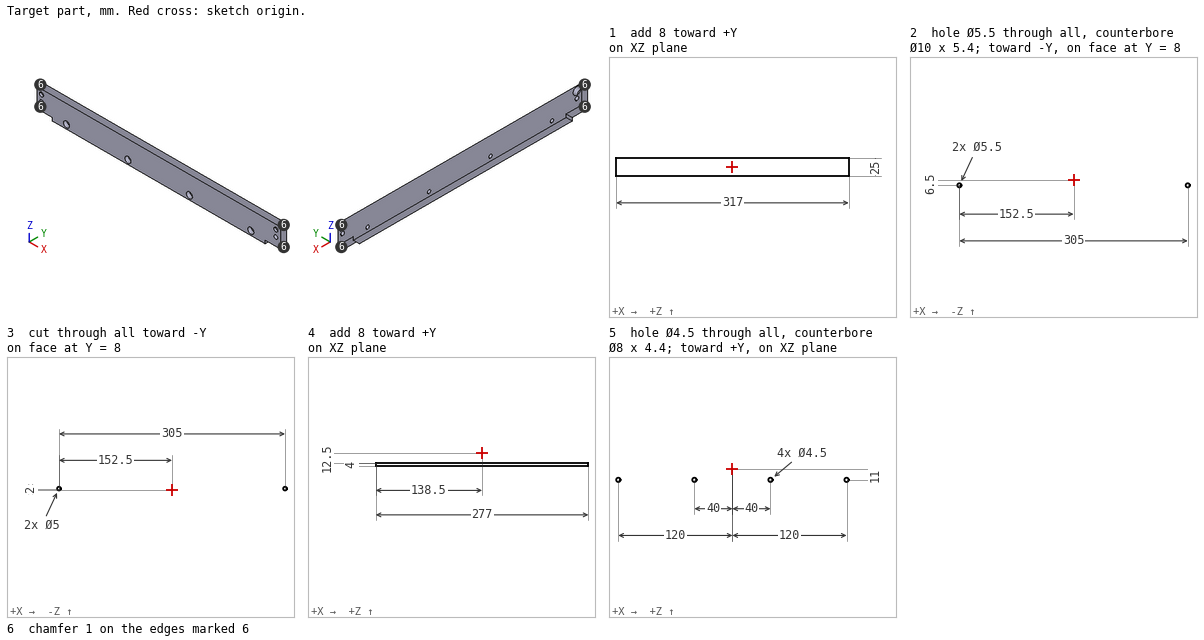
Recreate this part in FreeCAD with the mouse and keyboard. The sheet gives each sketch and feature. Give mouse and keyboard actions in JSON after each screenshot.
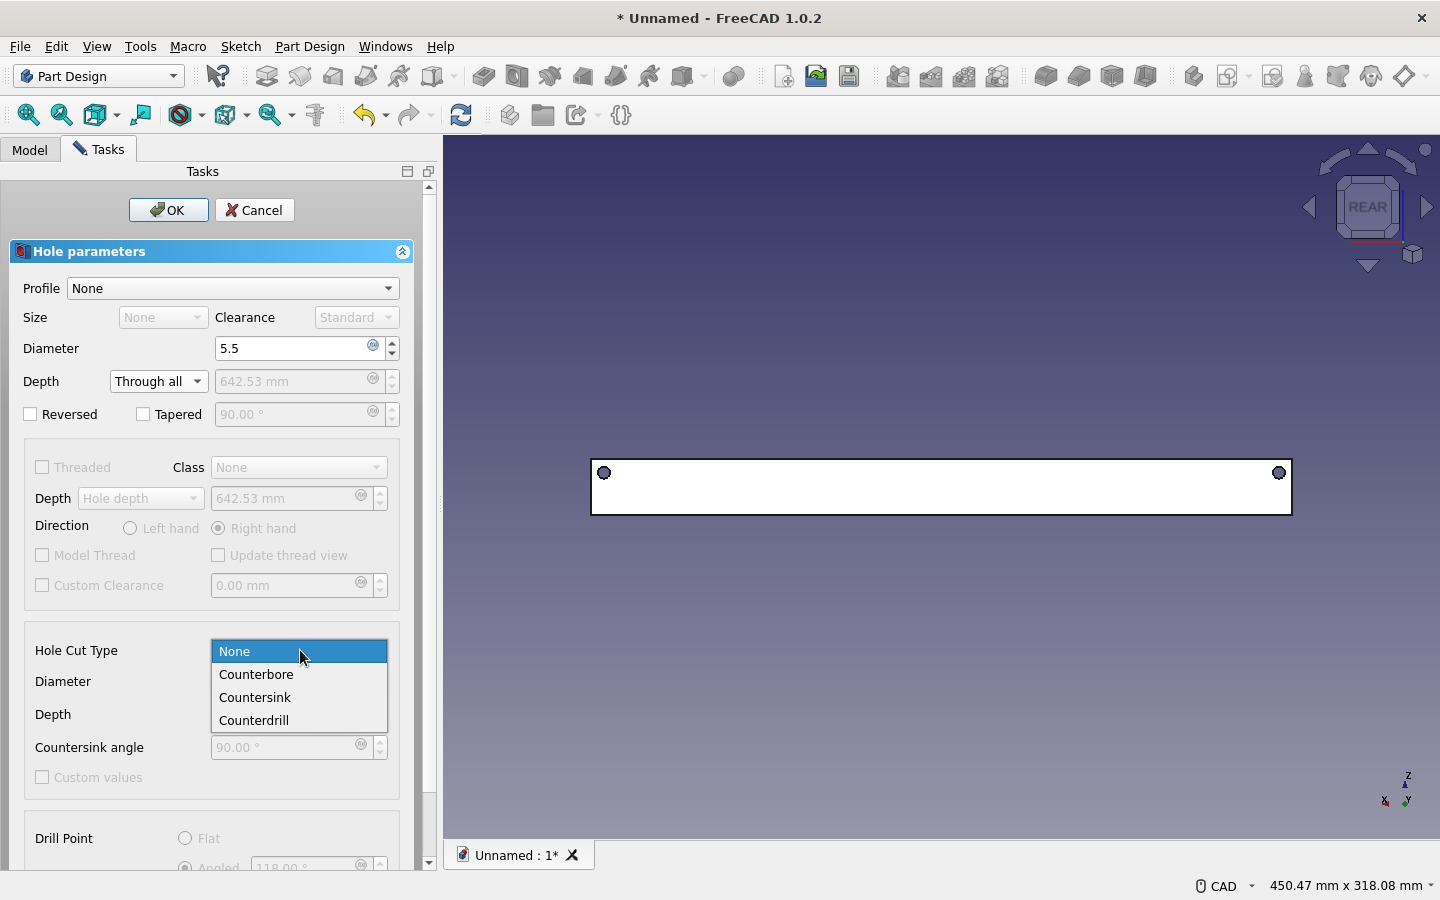
{"action": "left_click", "coordinate": [298, 674]}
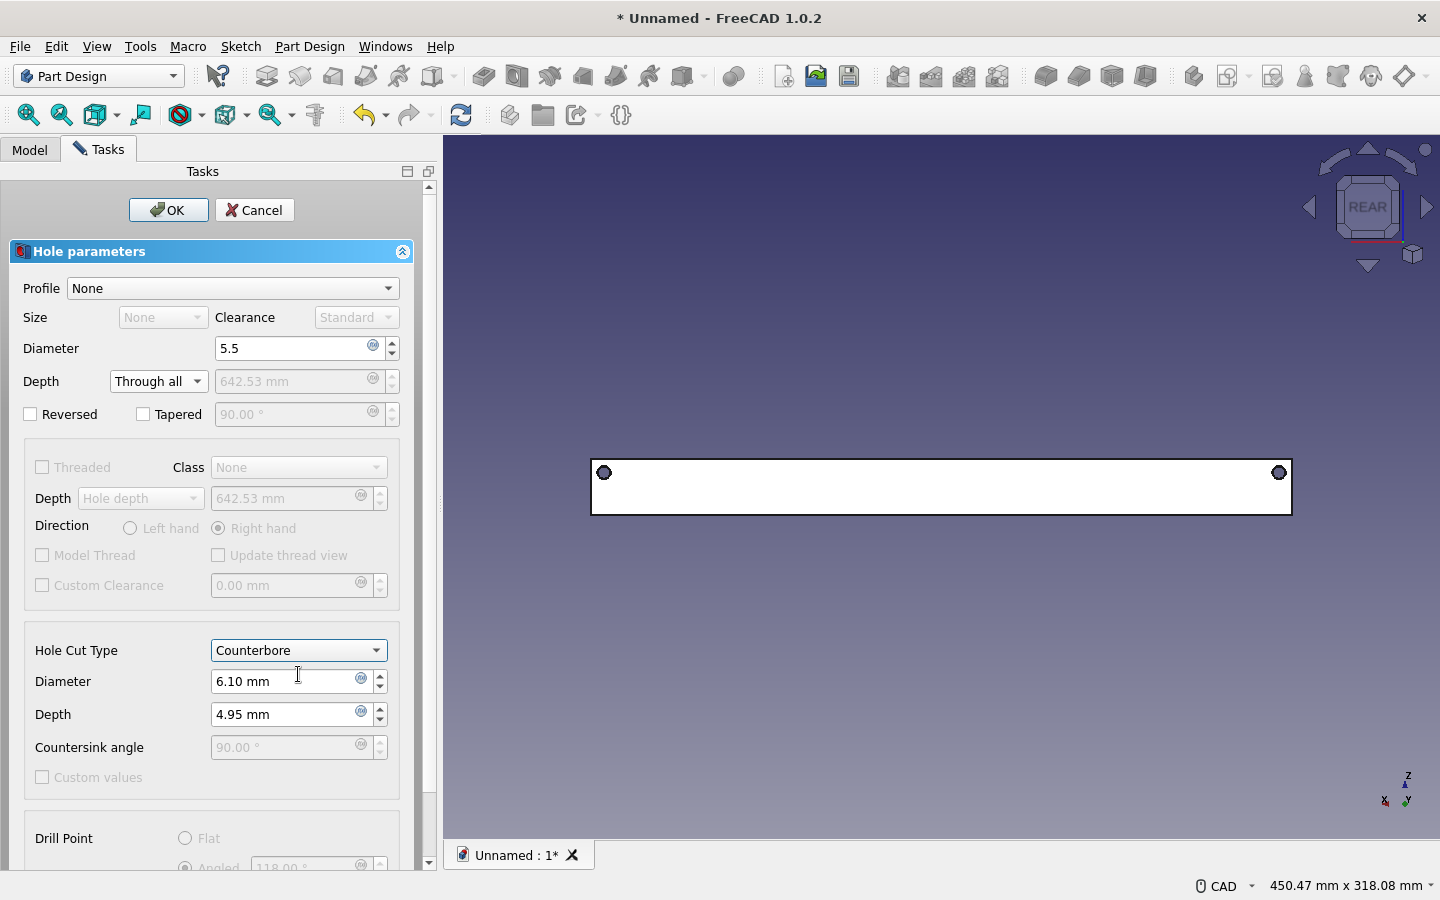
{"action": "triple_click", "coordinate": [292, 682]}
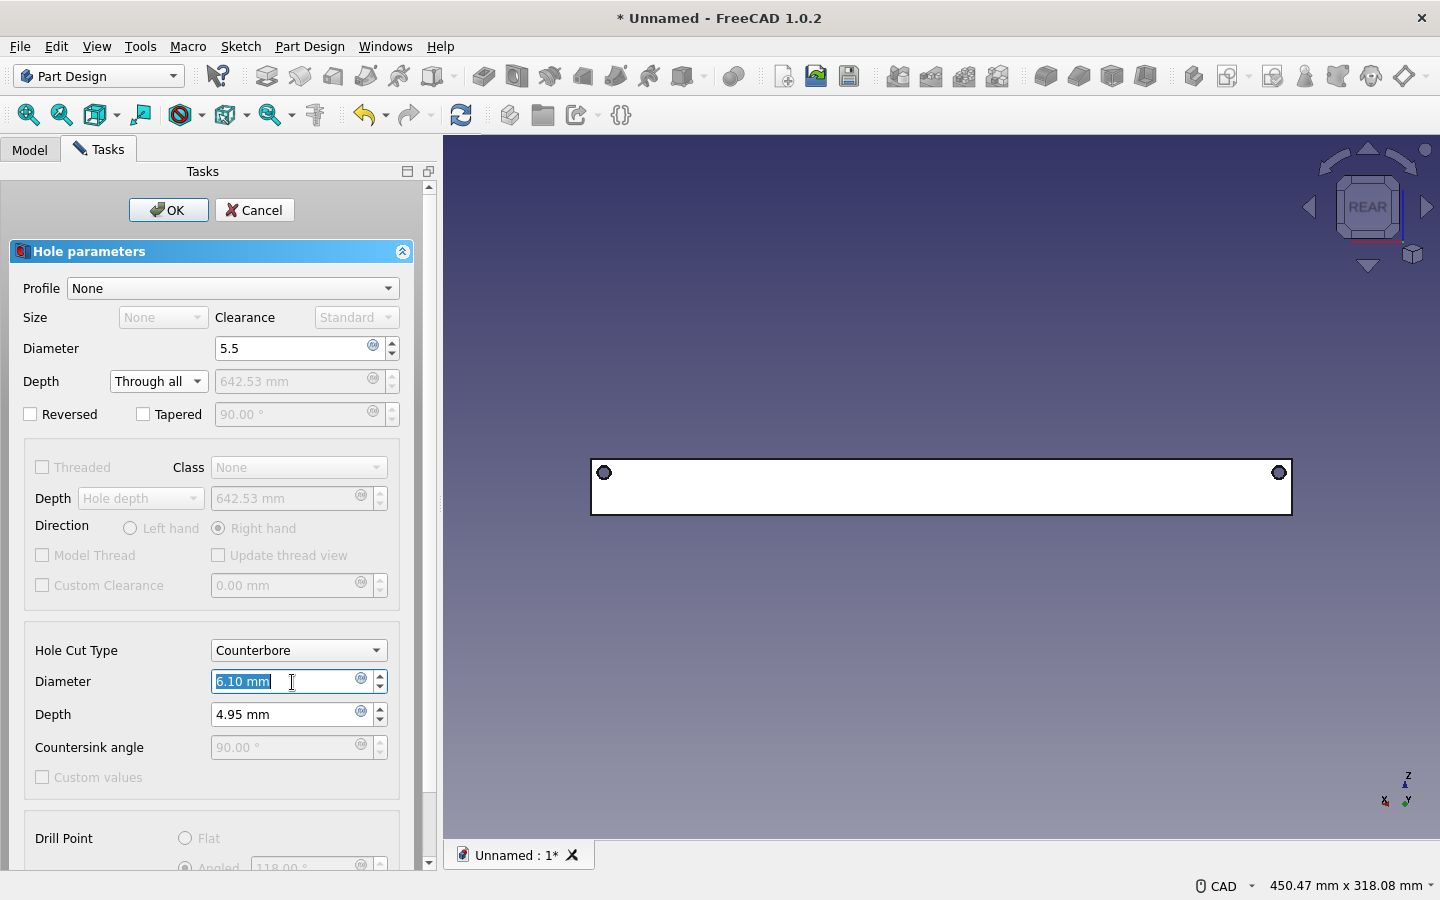
{"action": "type", "text": "10"}
{"action": "key", "text": "Tab"}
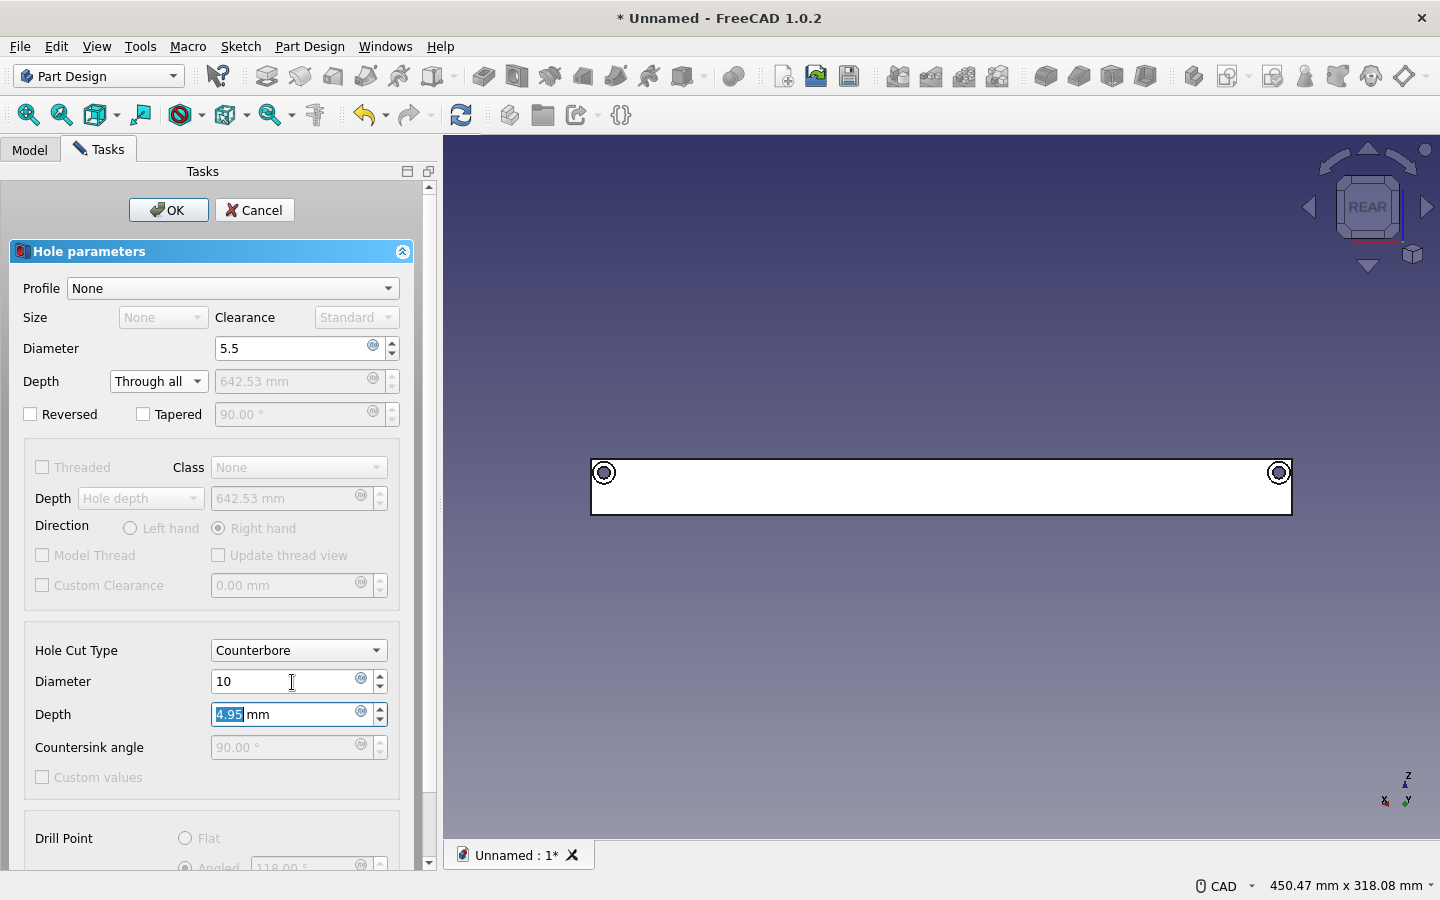
{"action": "type", "text": "5.4"}
{"action": "key", "text": "Tab"}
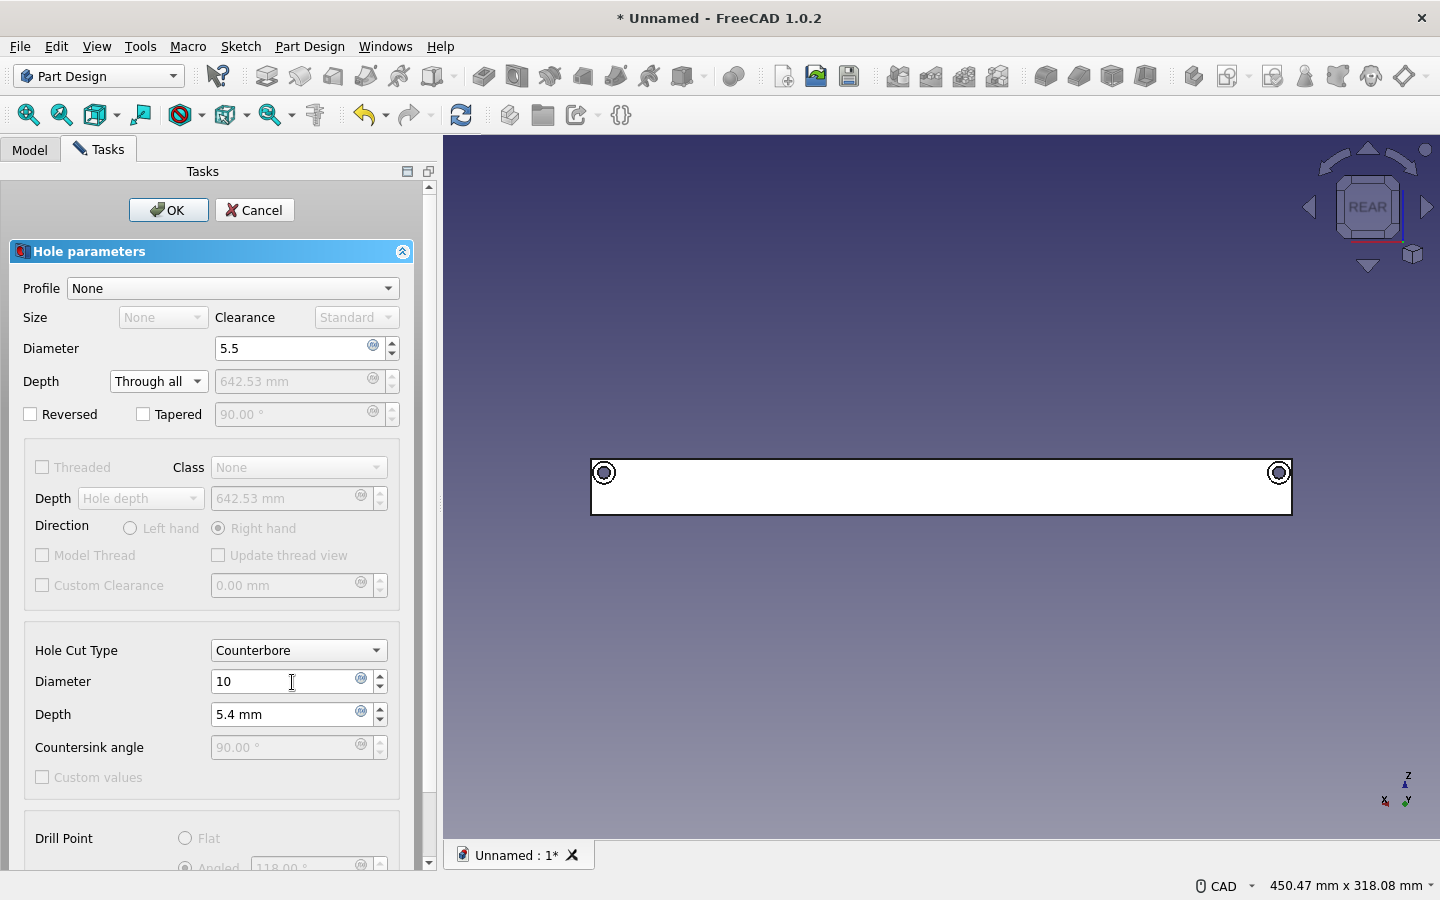
{"action": "left_click", "coordinate": [169, 210]}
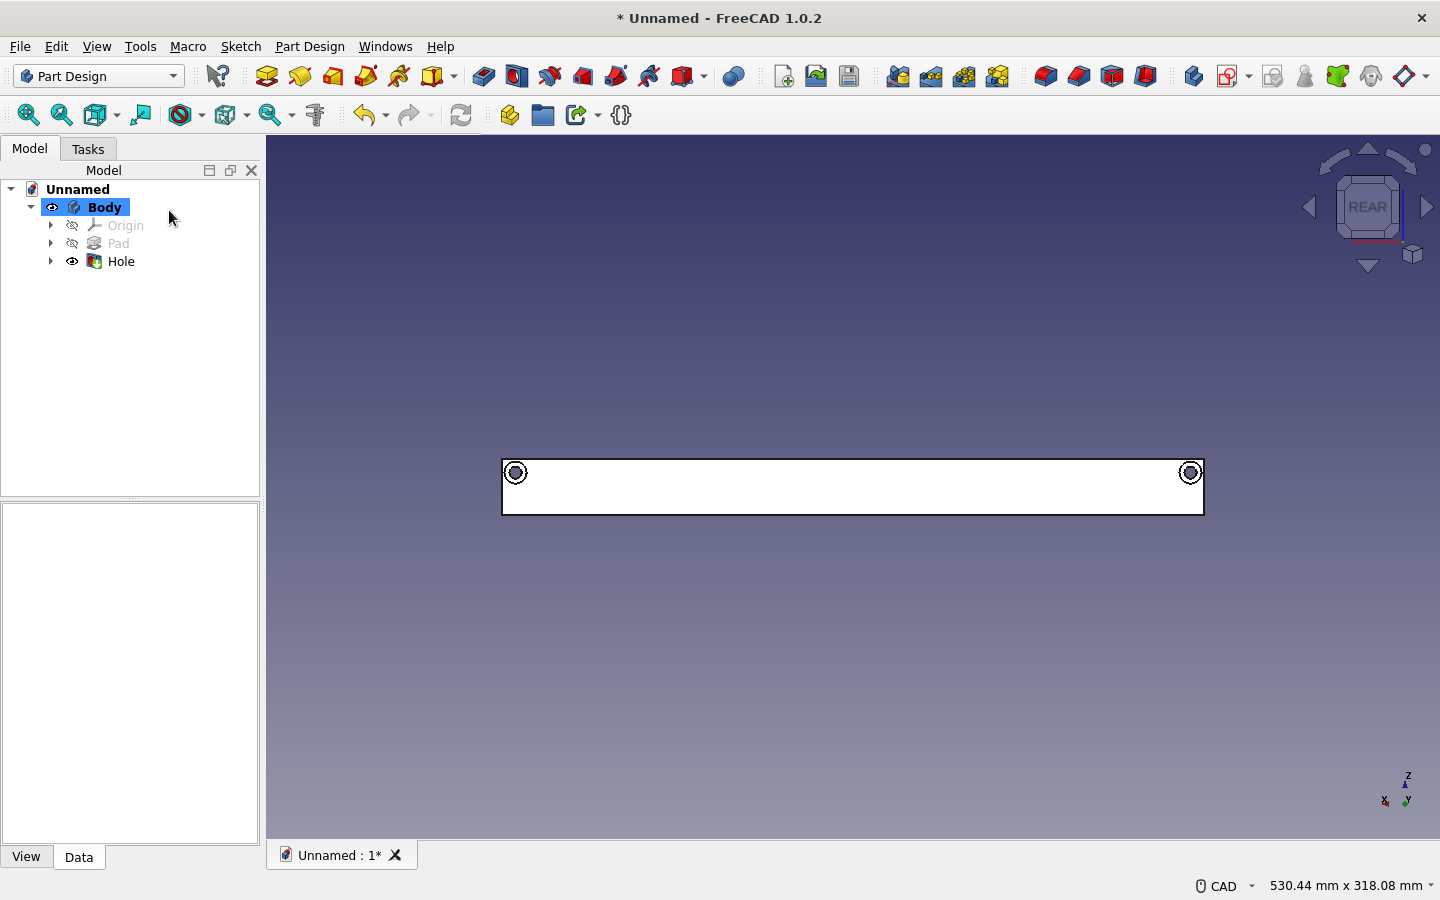
{"action": "left_click", "coordinate": [552, 486]}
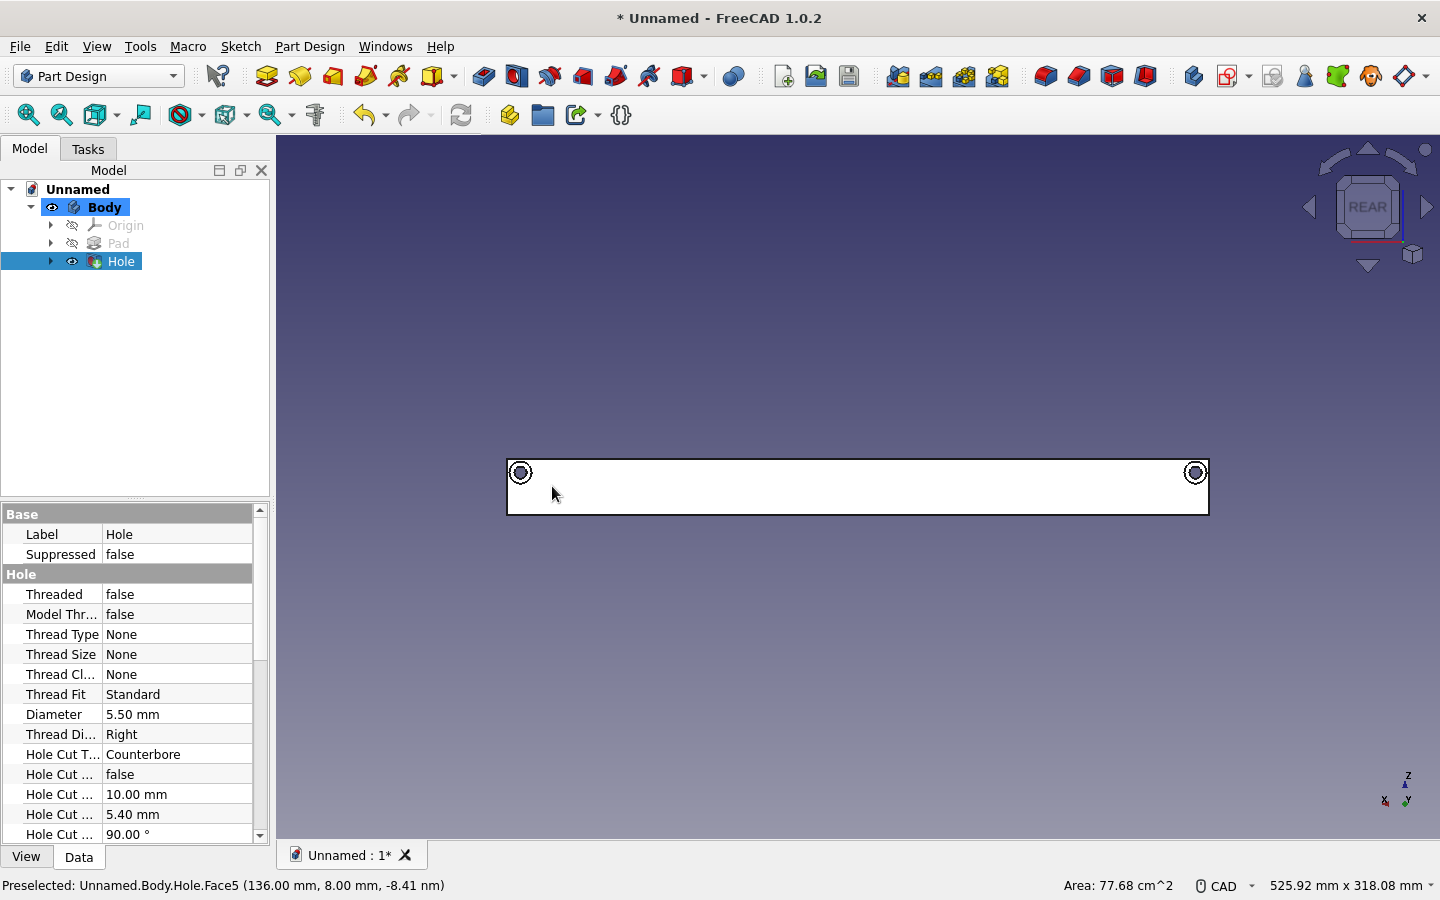
{"action": "left_click", "coordinate": [1226, 76]}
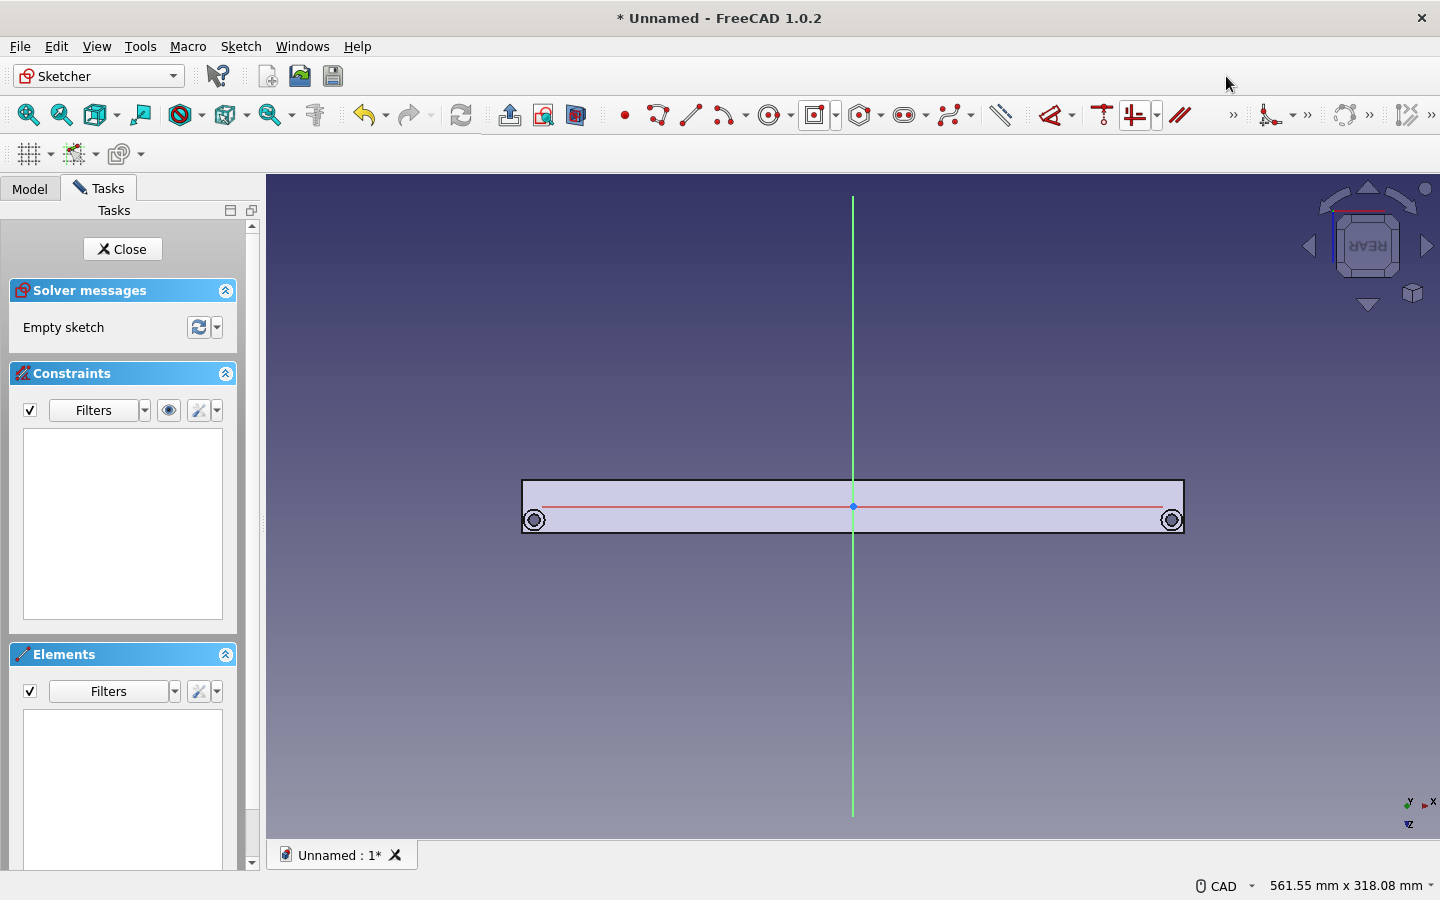
{"action": "left_click", "coordinate": [768, 116]}